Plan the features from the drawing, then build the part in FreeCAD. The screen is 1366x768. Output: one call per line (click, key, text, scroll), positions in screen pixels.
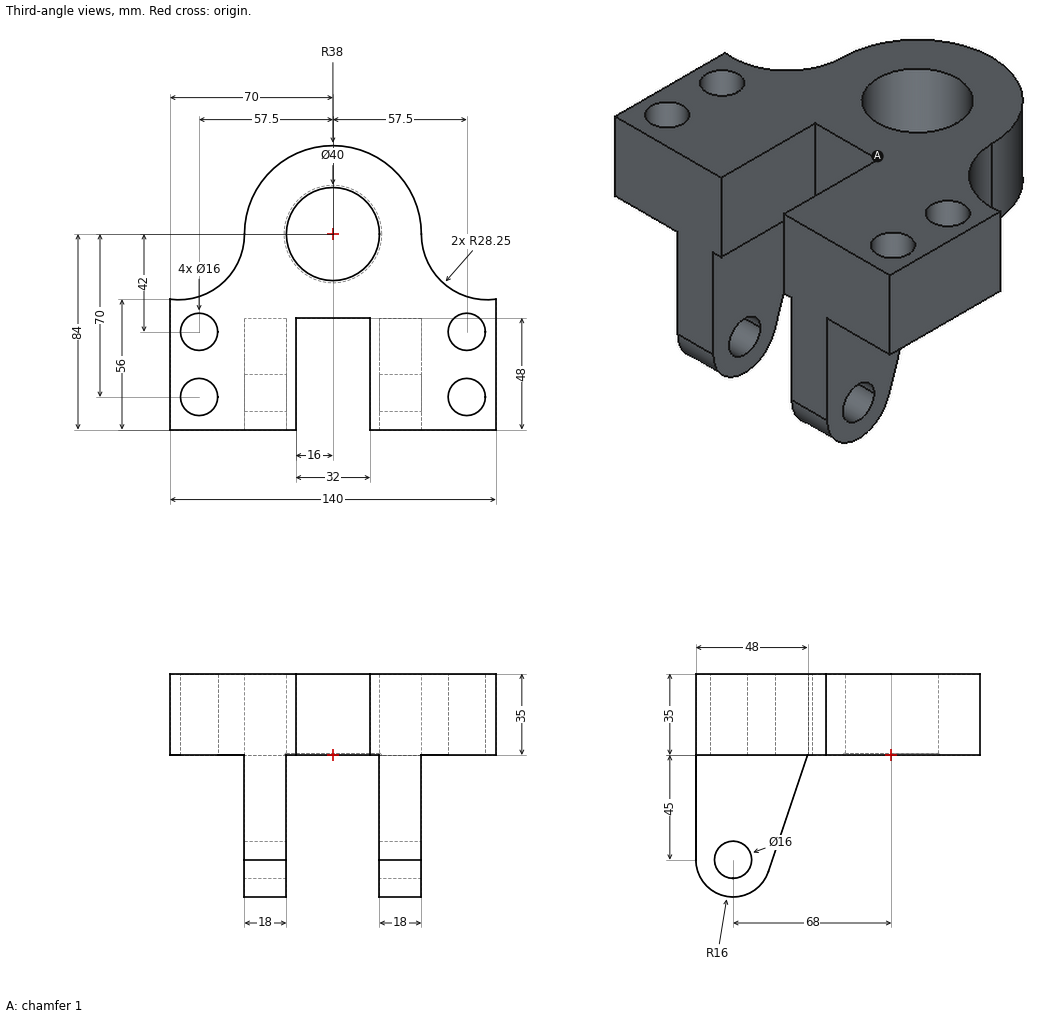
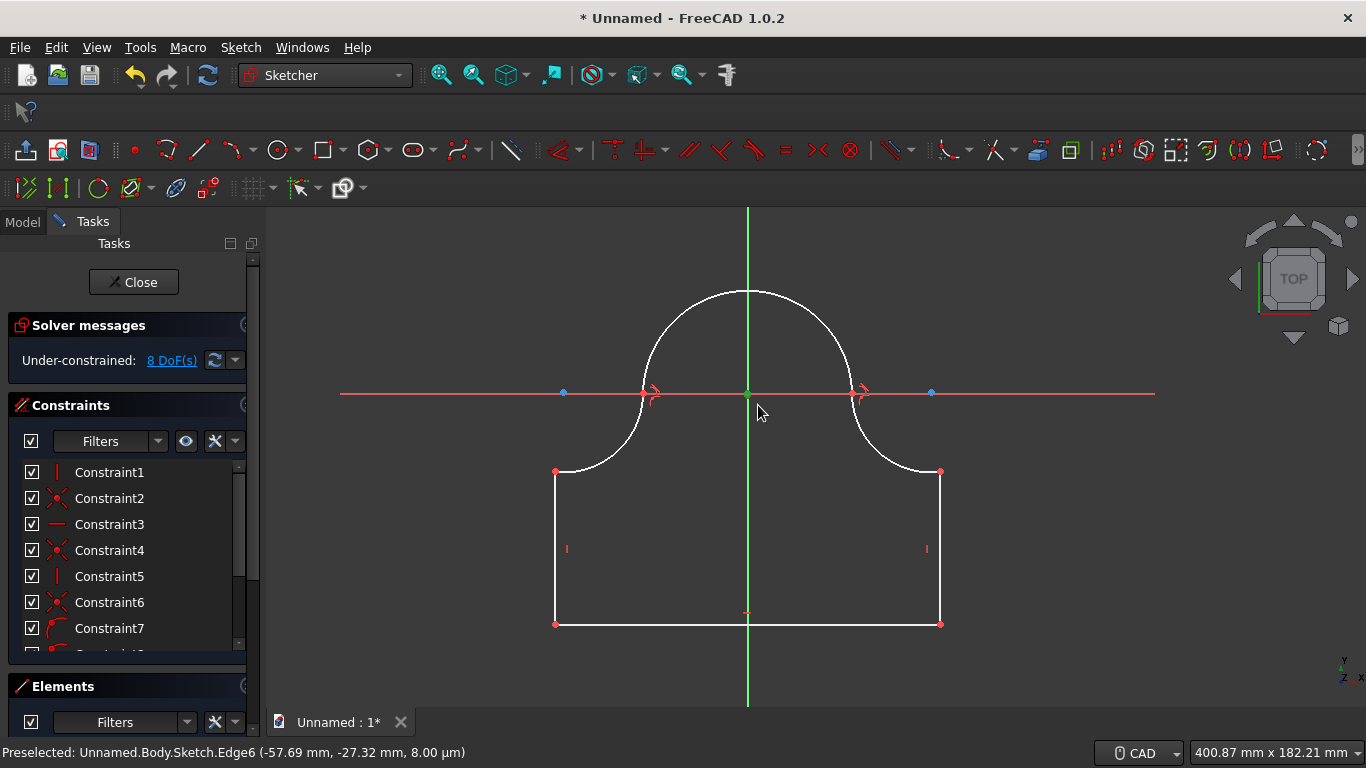
key(c)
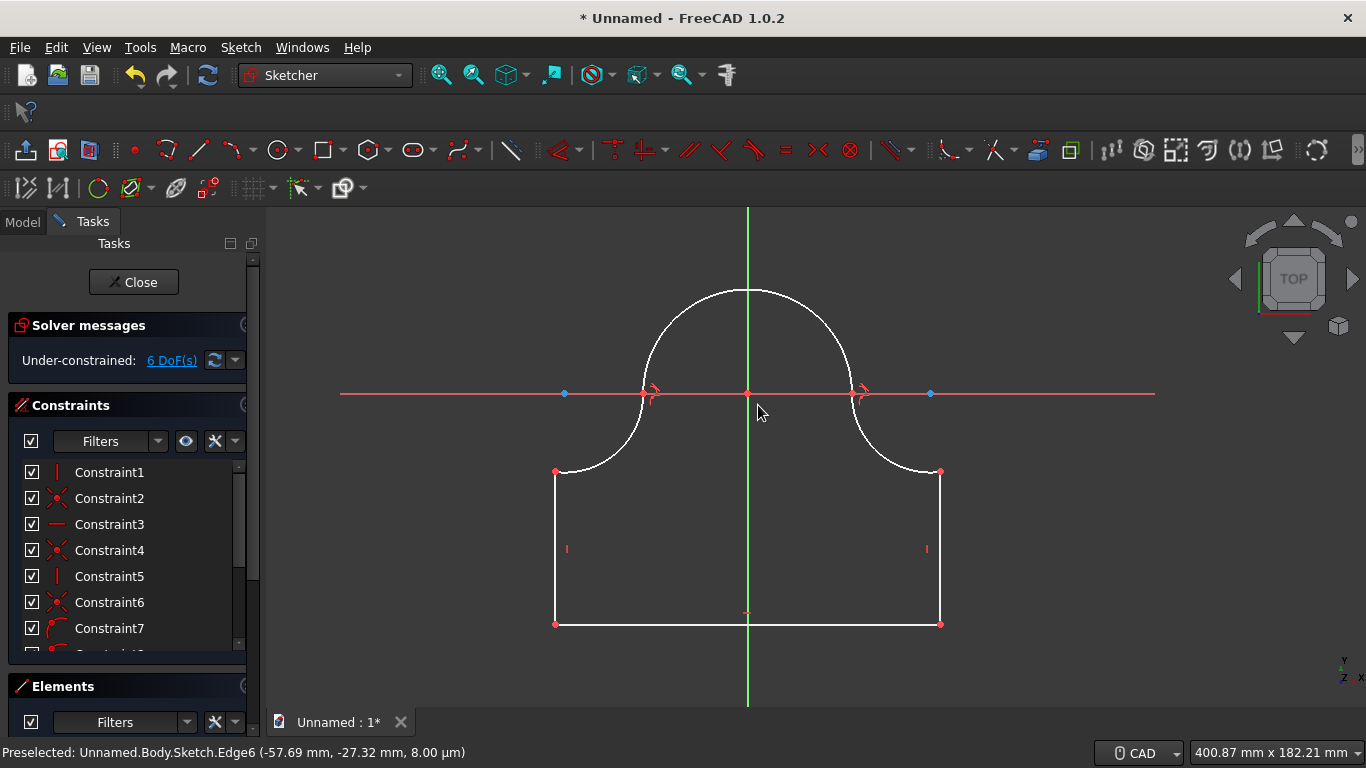
click(862, 432)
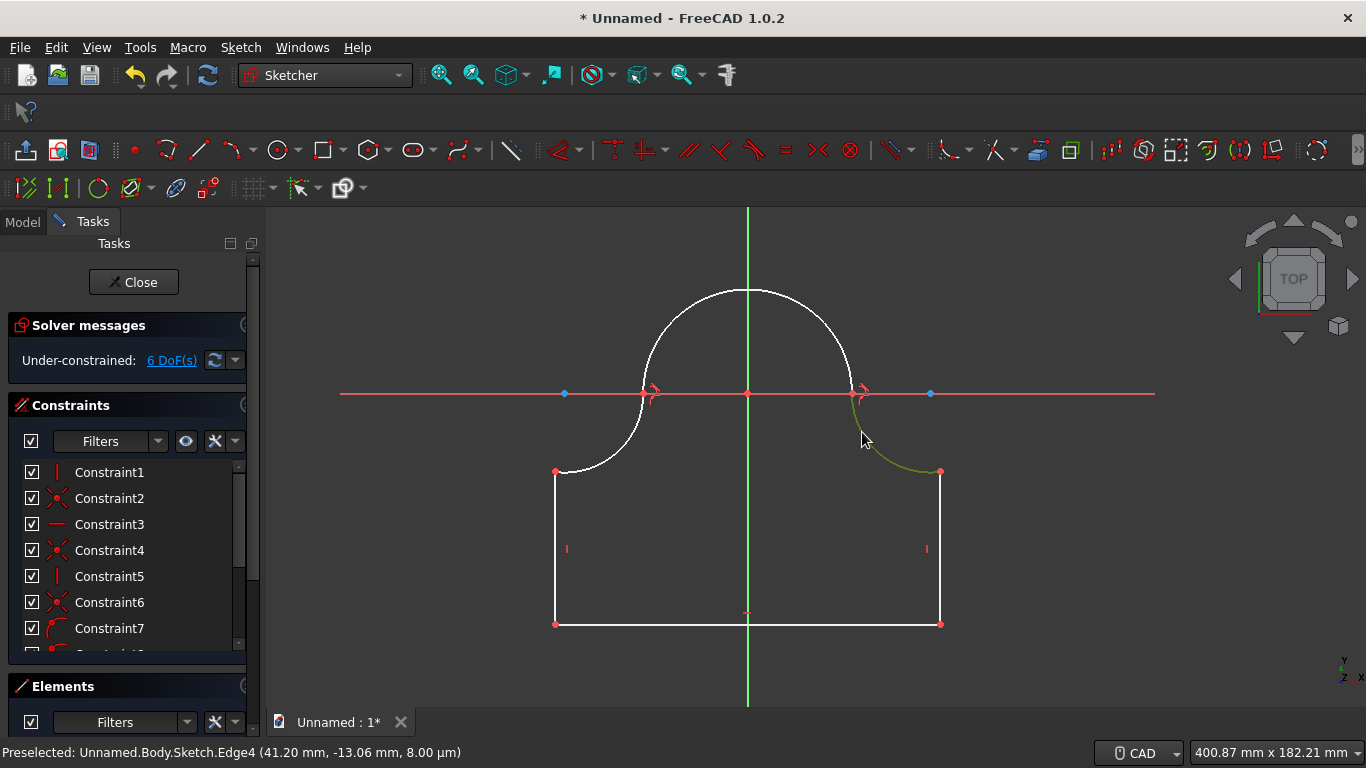
click(594, 467)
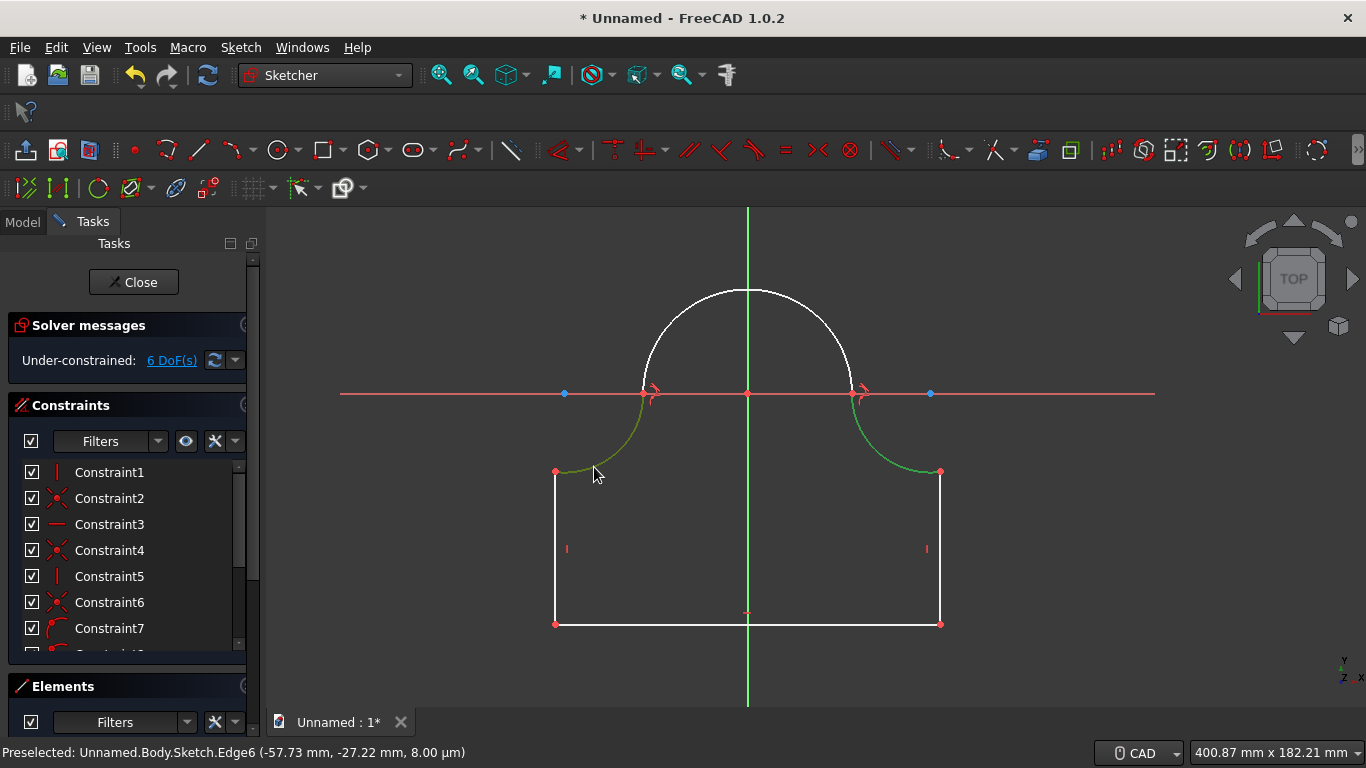
key(e)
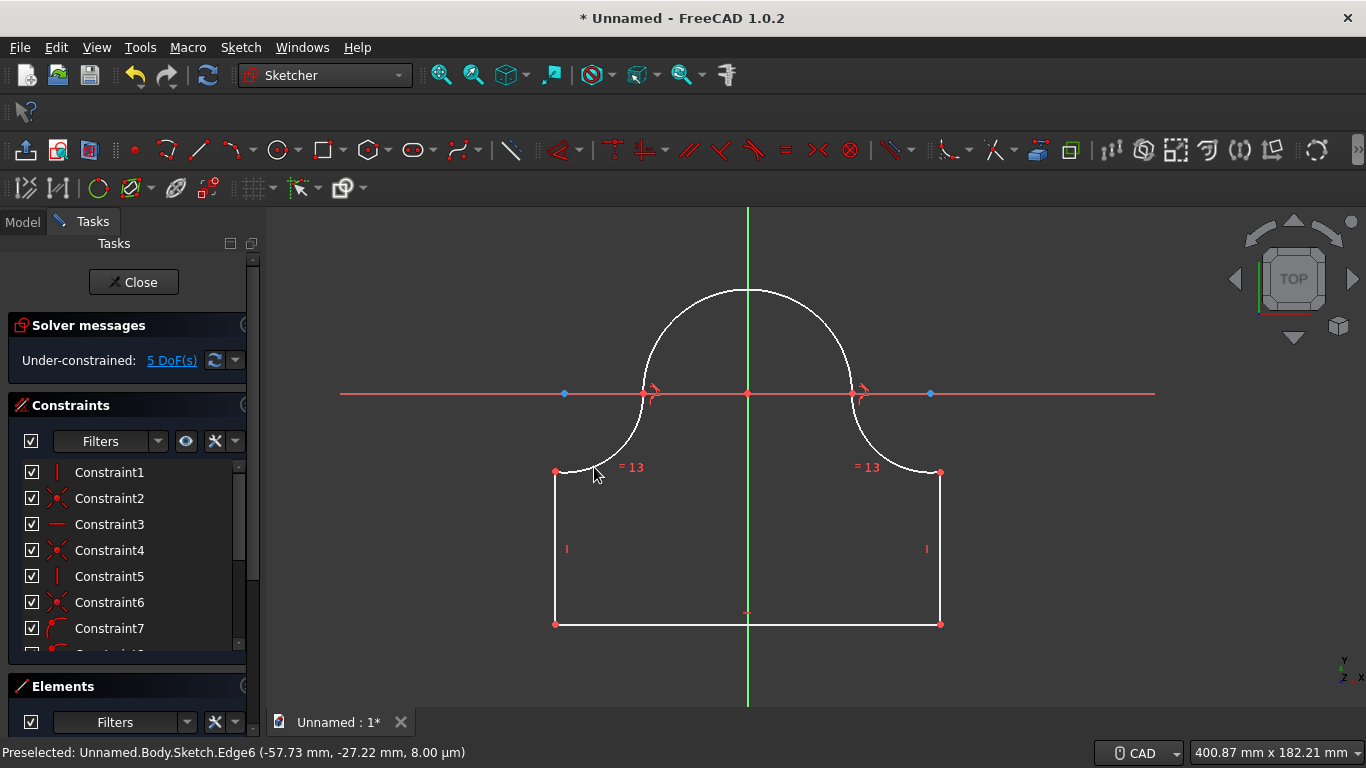
key(d)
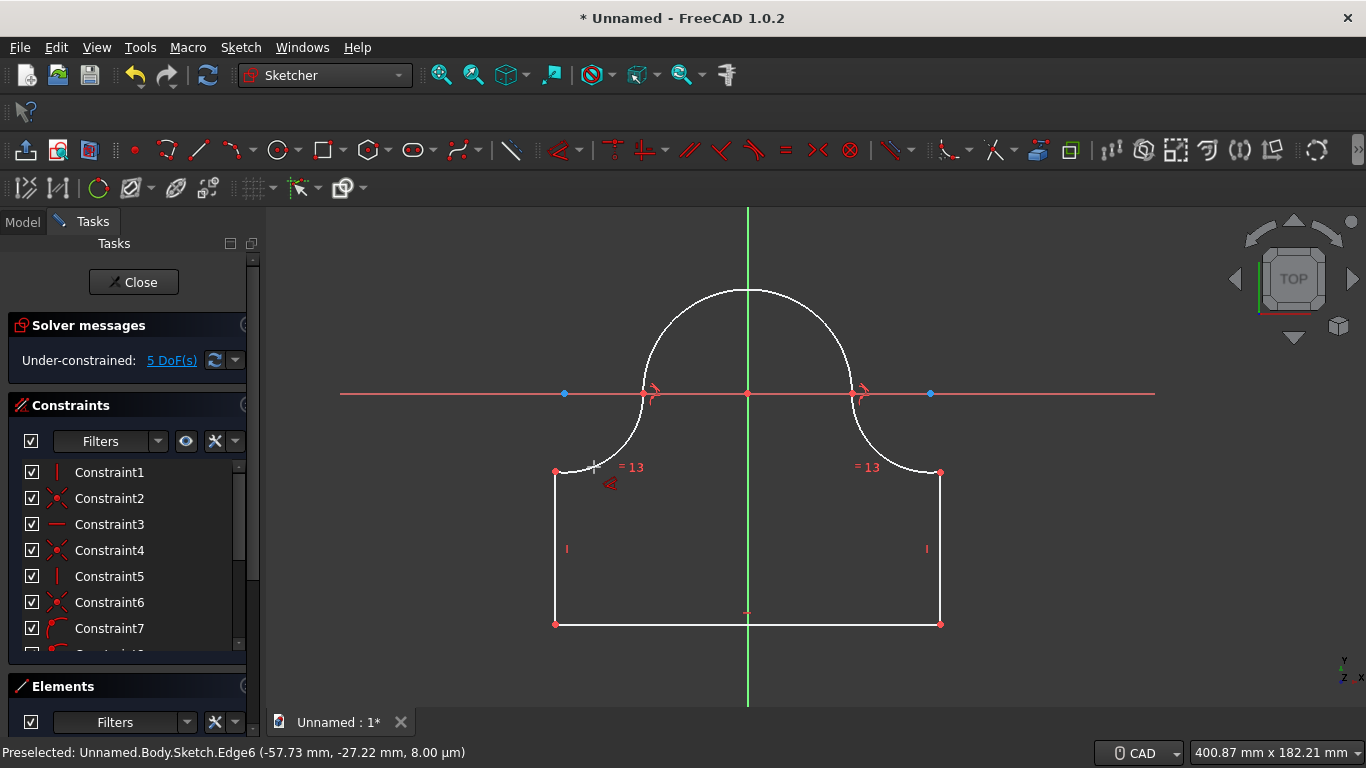
click(862, 432)
click(834, 448)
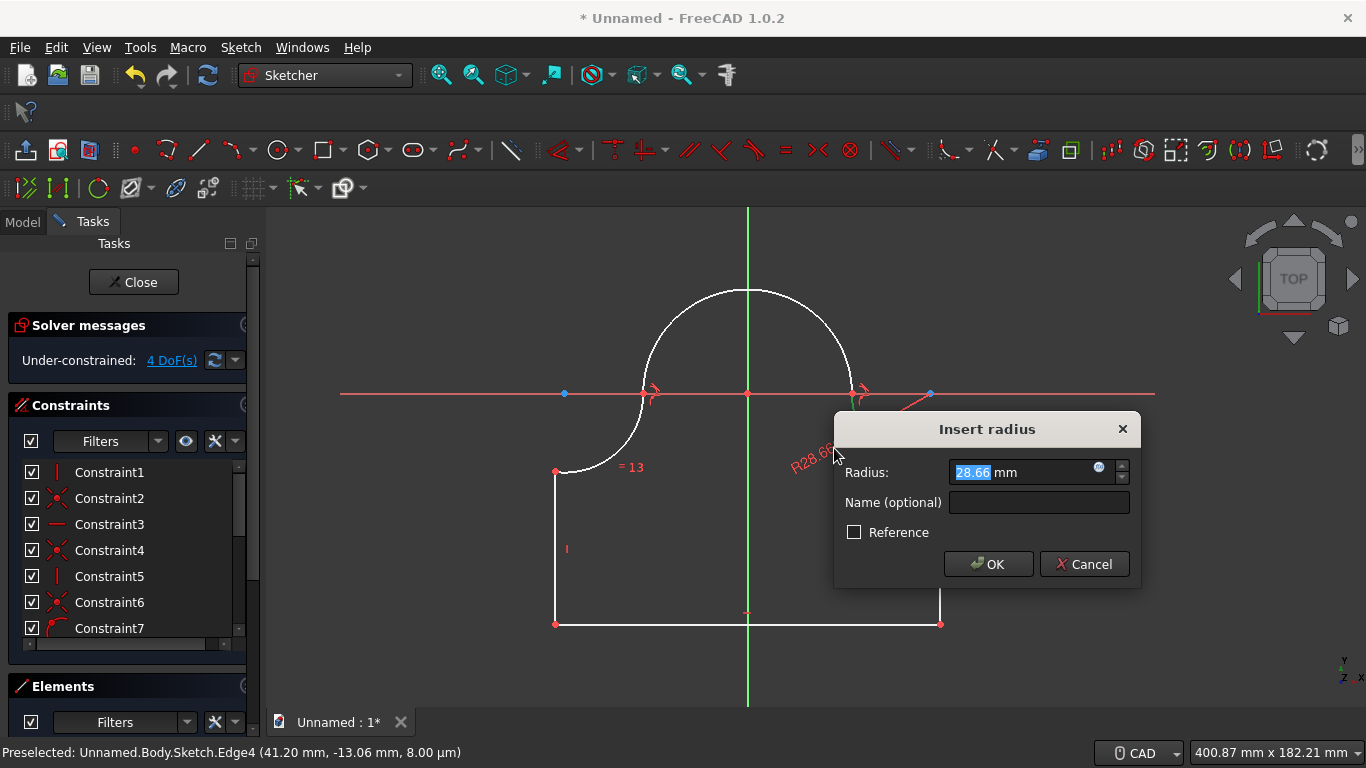
text(28.25)
key(Return)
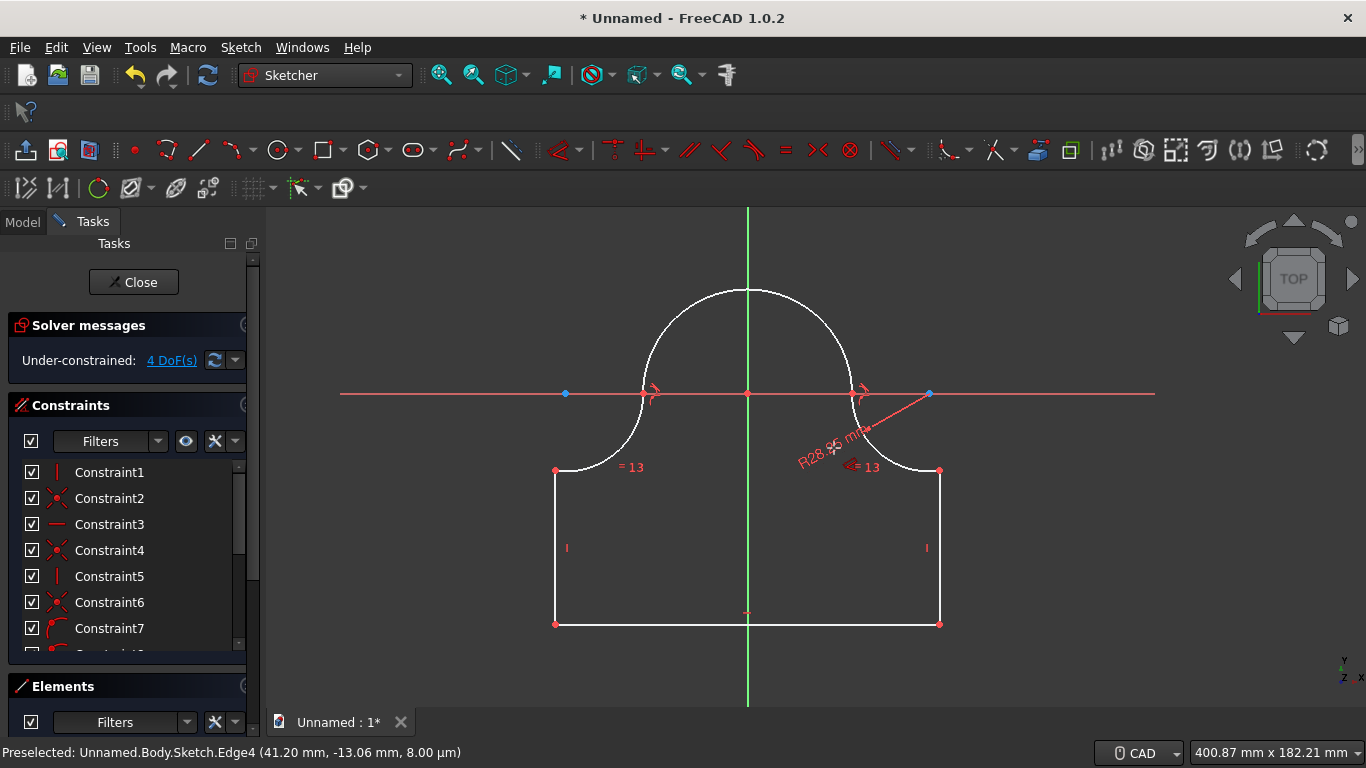
click(809, 309)
click(828, 283)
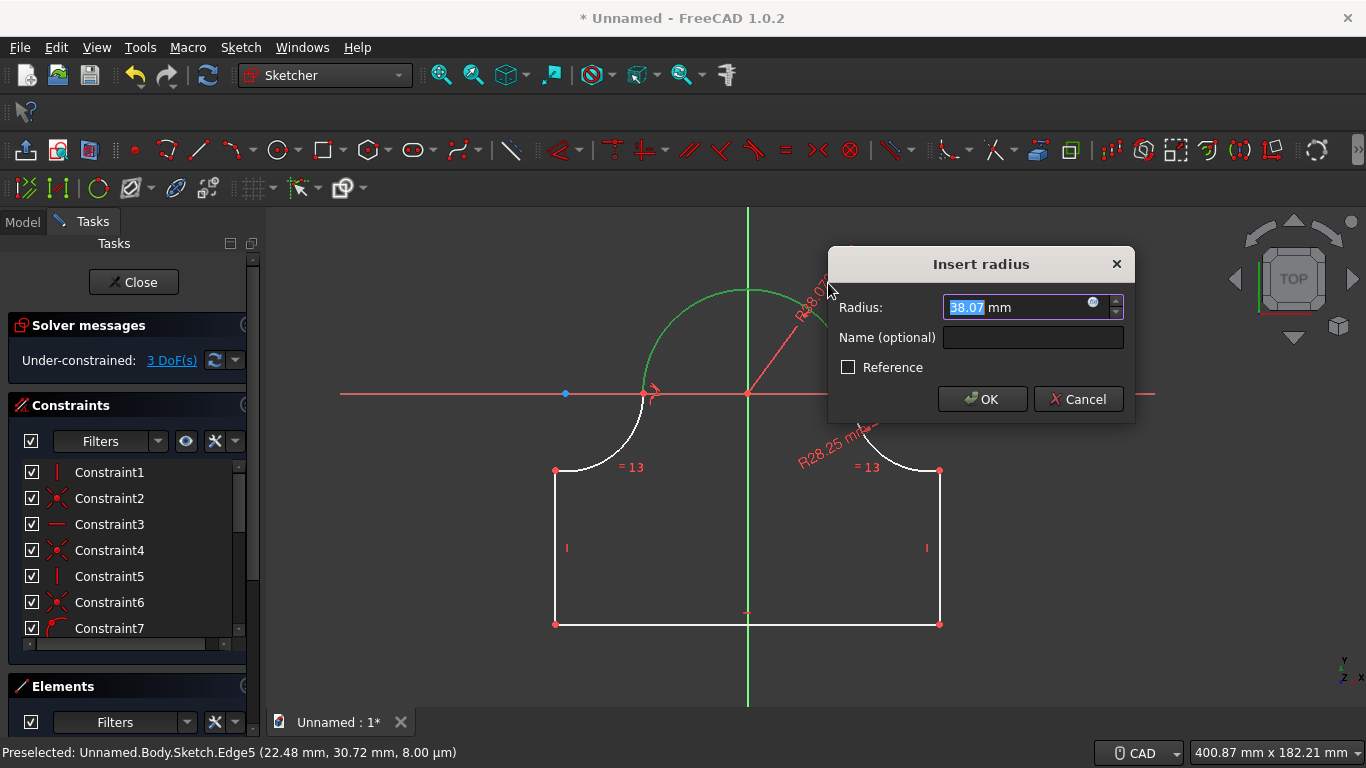
text(38)
key(Return)